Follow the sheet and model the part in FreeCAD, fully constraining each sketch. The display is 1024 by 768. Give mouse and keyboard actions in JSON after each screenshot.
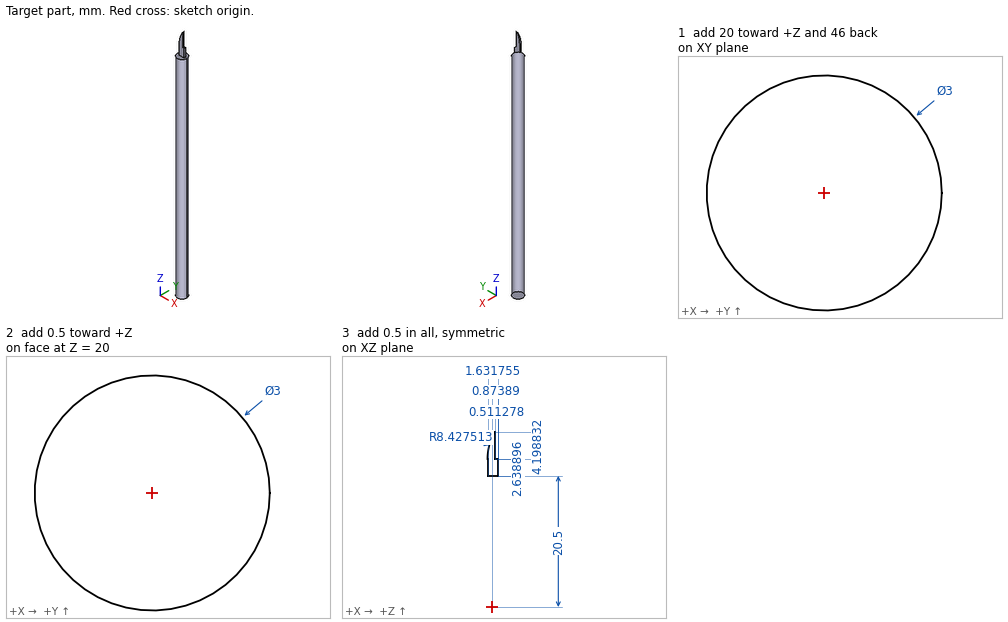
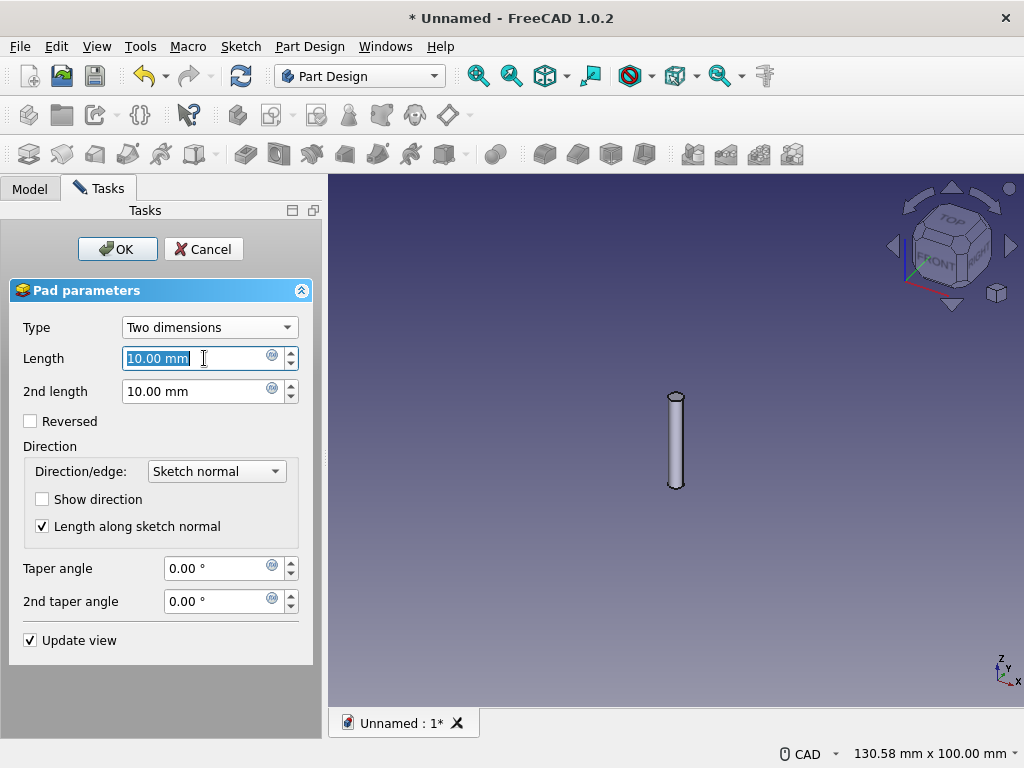
{"action": "type", "text": "20"}
{"action": "key", "text": "Tab"}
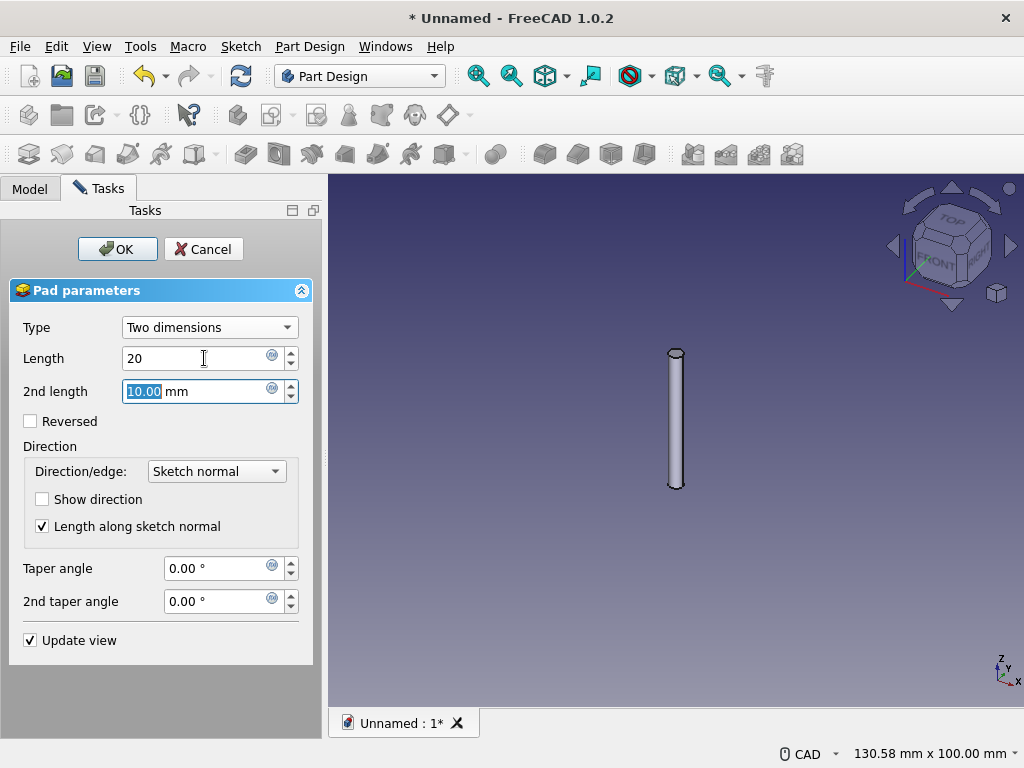
{"action": "type", "text": "46"}
{"action": "key", "text": "Tab"}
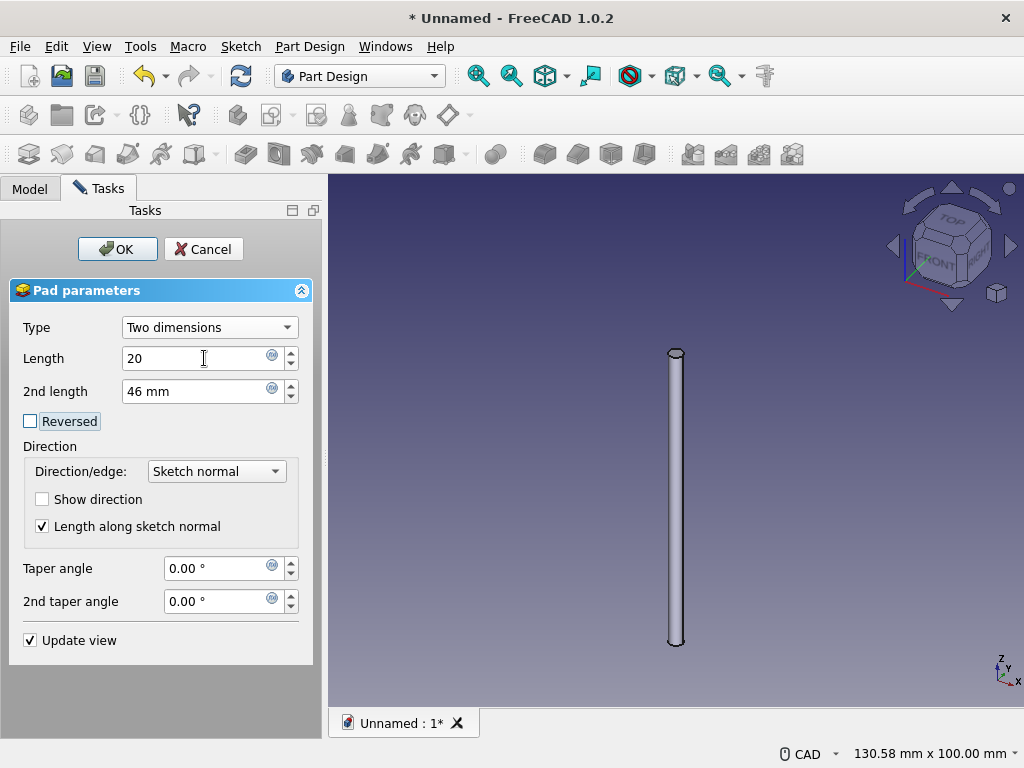
{"action": "left_click", "coordinate": [118, 249]}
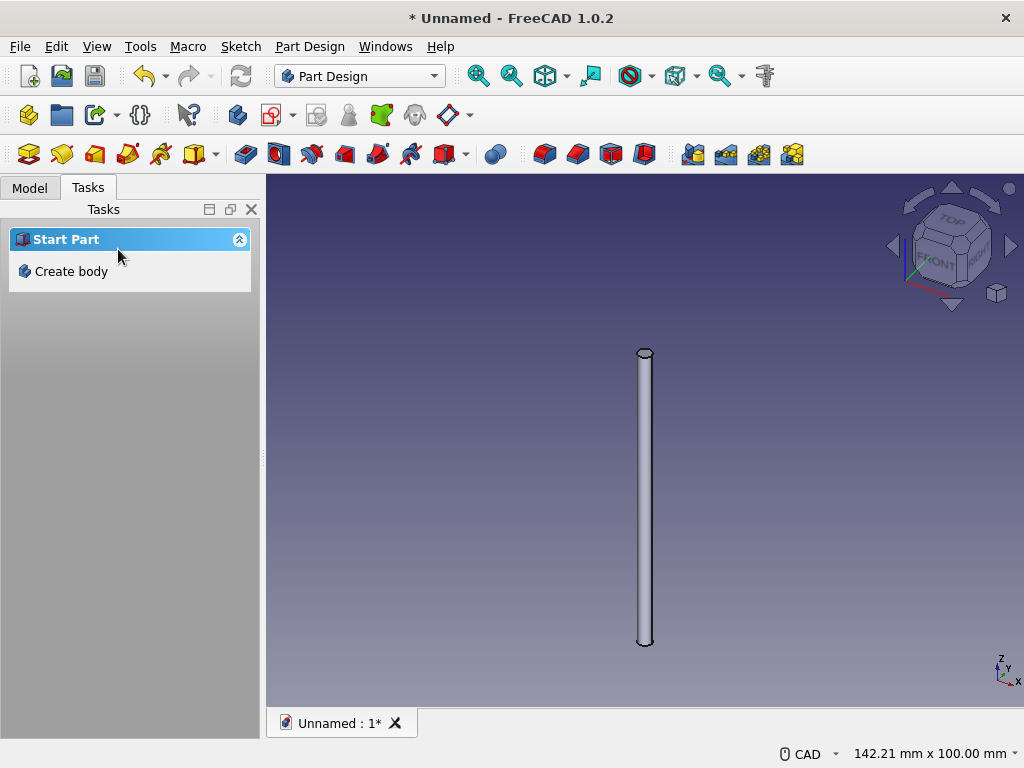
{"action": "key", "text": "0"}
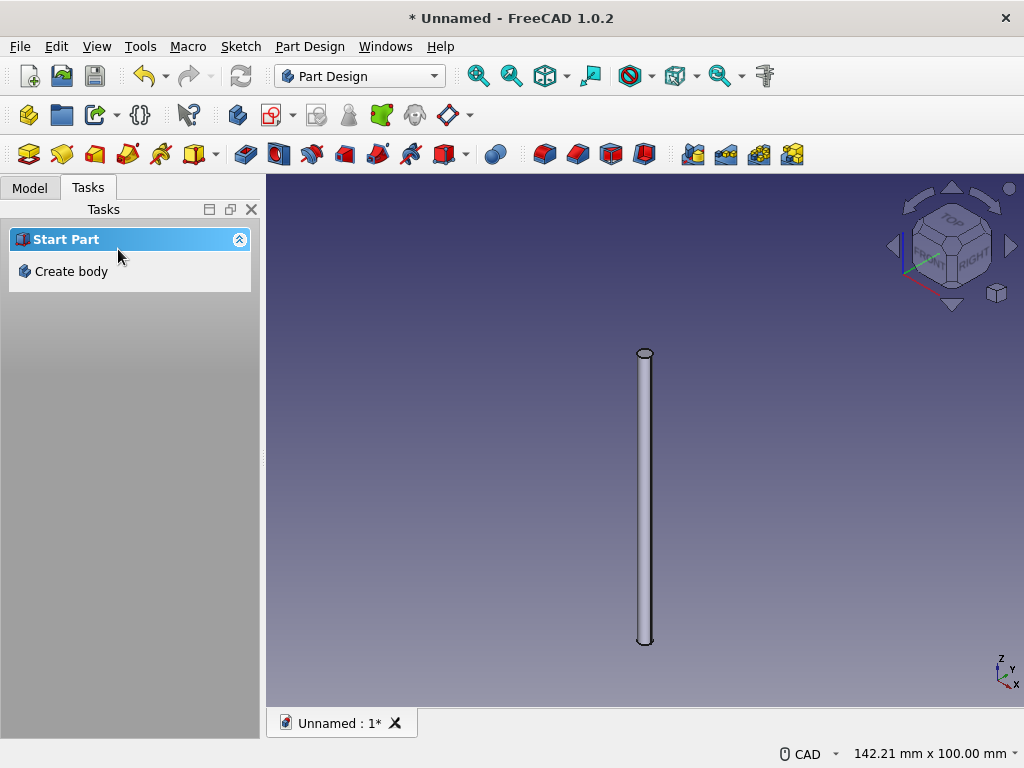
{"action": "key", "text": "2"}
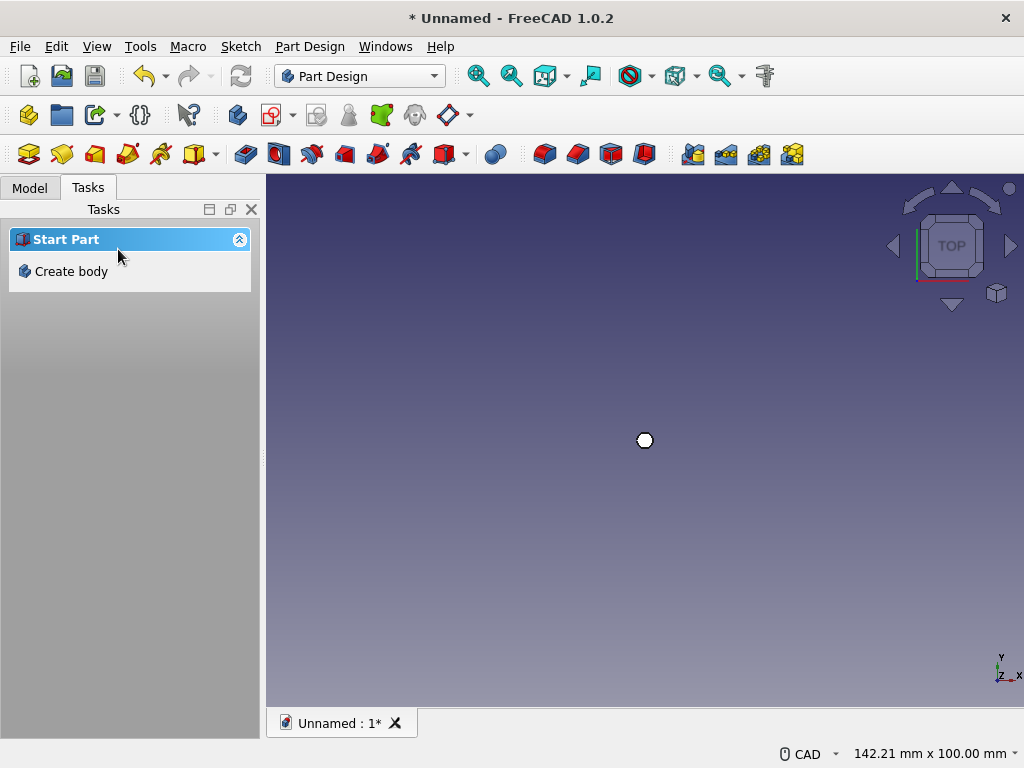
{"action": "left_click", "coordinate": [479, 76]}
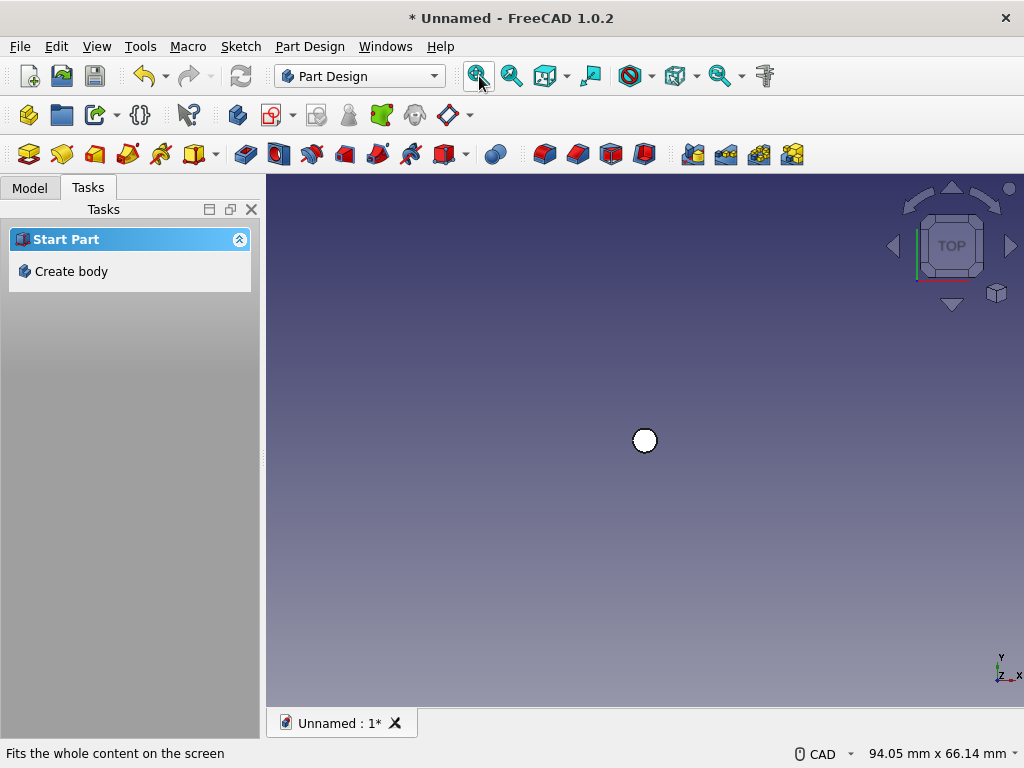
{"action": "left_click", "coordinate": [645, 439]}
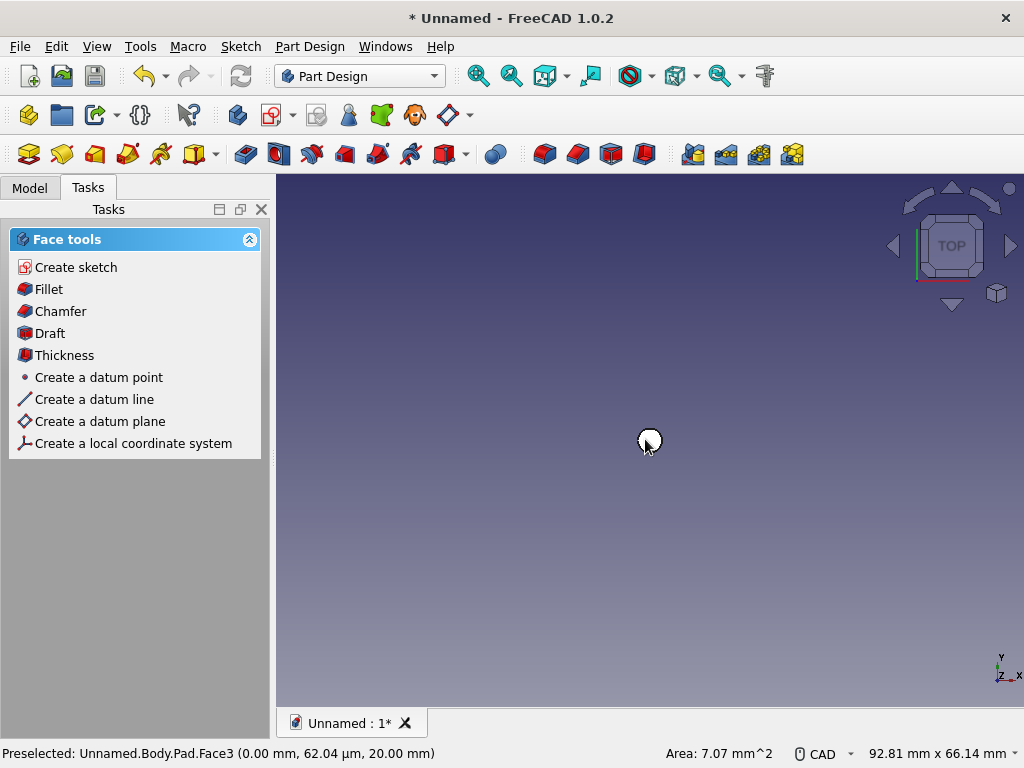
{"action": "left_click", "coordinate": [270, 116]}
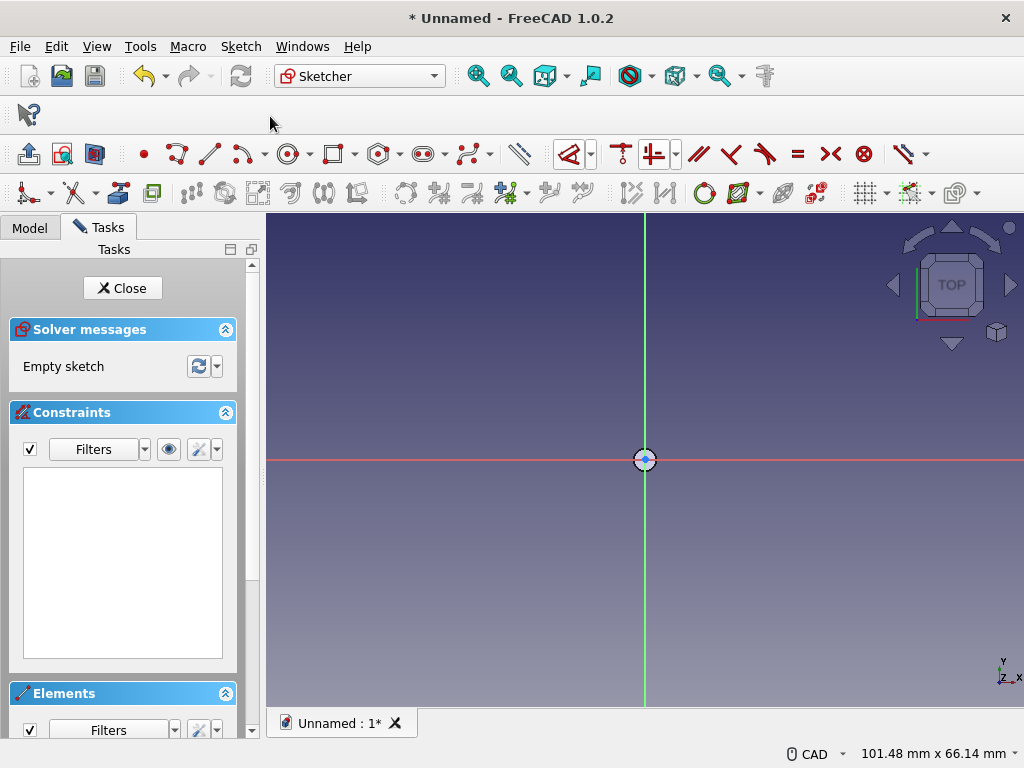
{"action": "scroll", "coordinate": [650, 460], "scroll_direction": "up", "scroll_amount": 13}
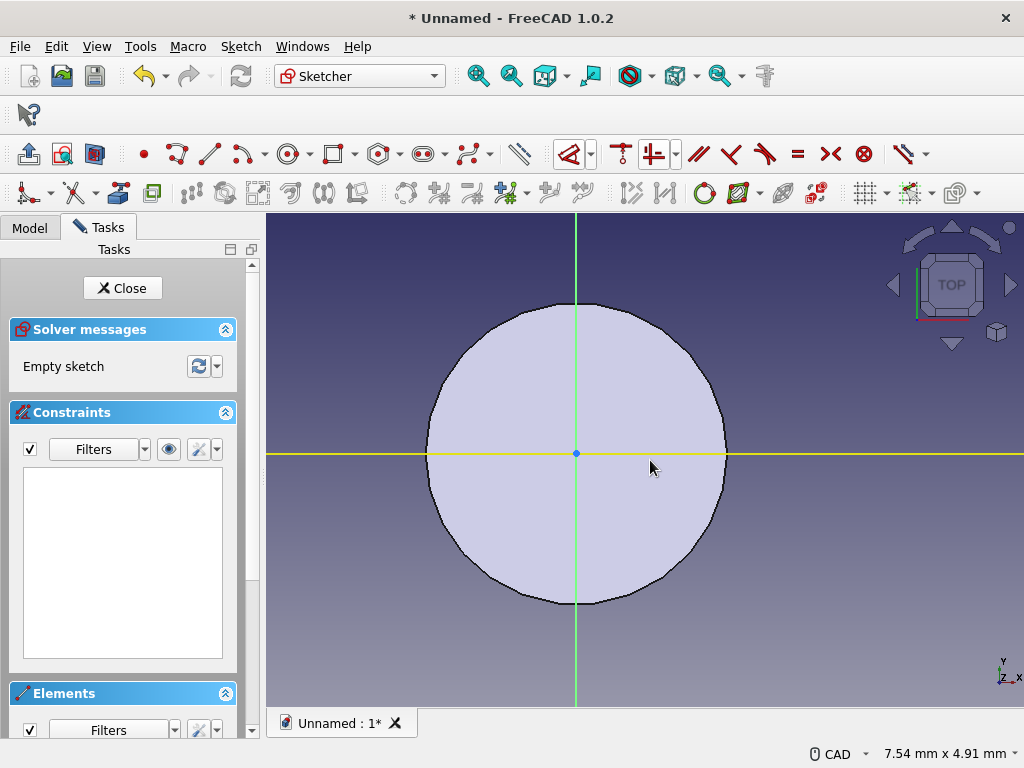
{"action": "left_click", "coordinate": [288, 154]}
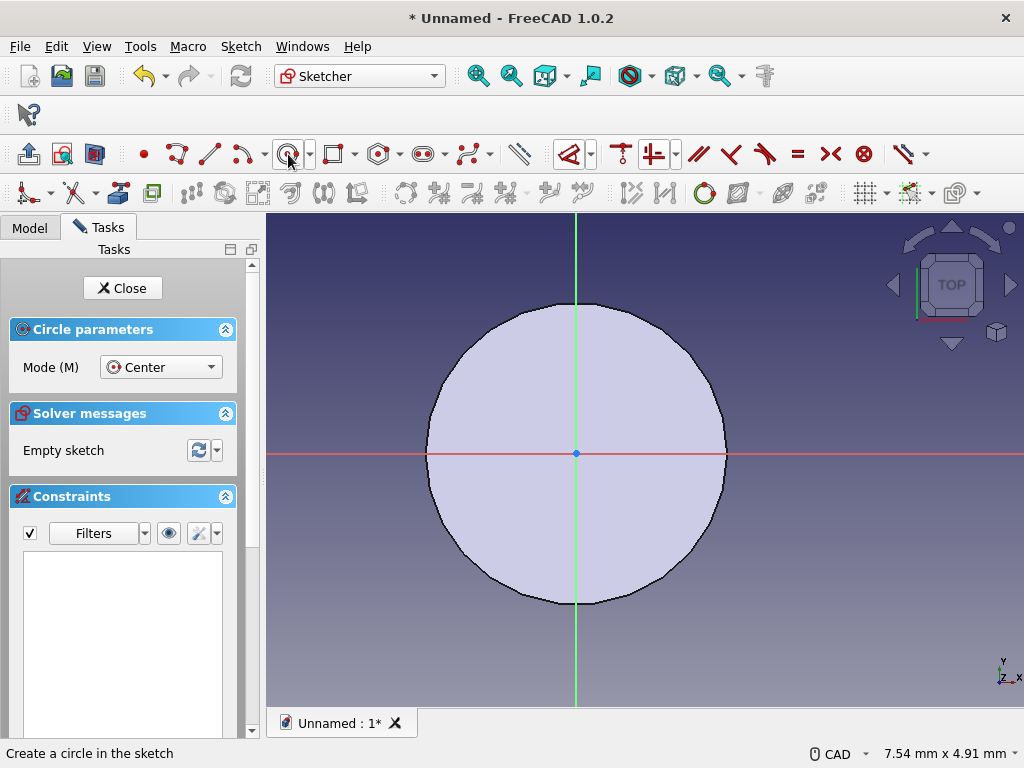
{"action": "left_click", "coordinate": [576, 454]}
{"action": "mouse_move", "coordinate": [683, 347]}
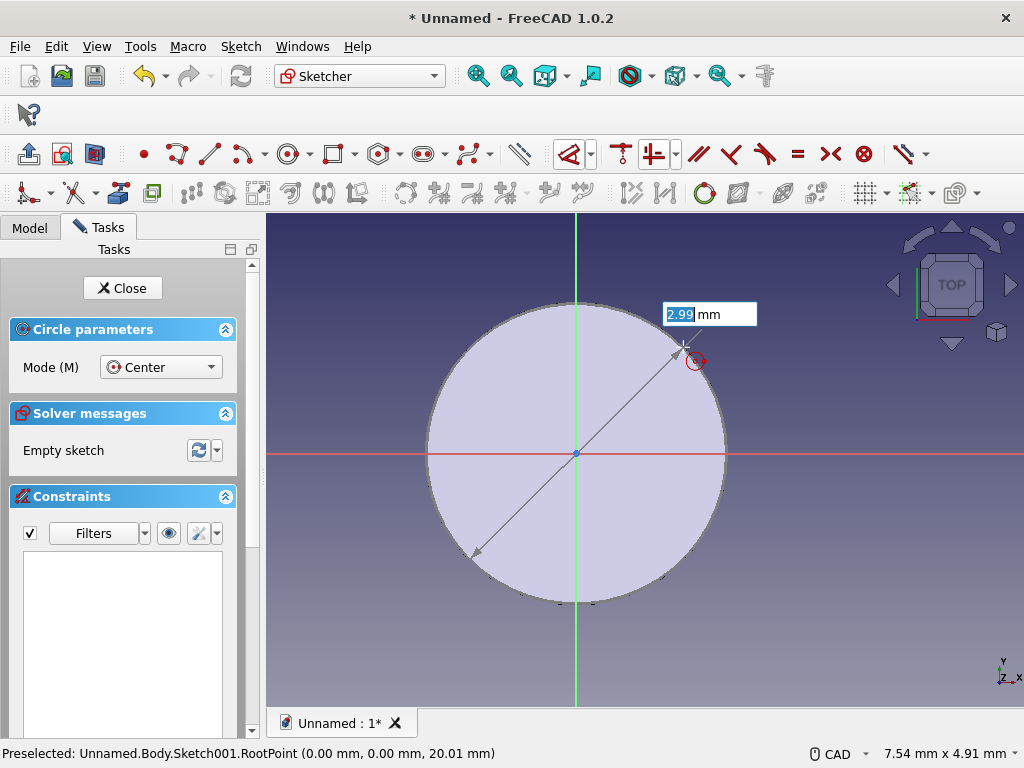
{"action": "type", "text": "3"}
{"action": "key", "text": "Return"}
{"action": "key", "text": "Escape"}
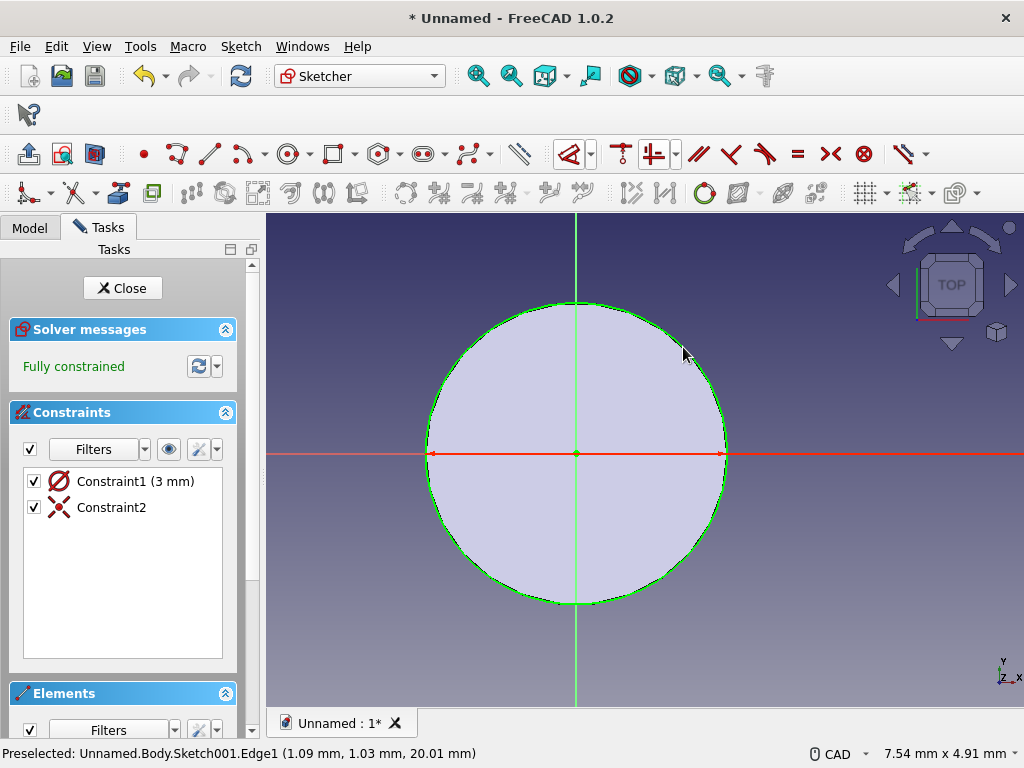
{"action": "left_click", "coordinate": [123, 288]}